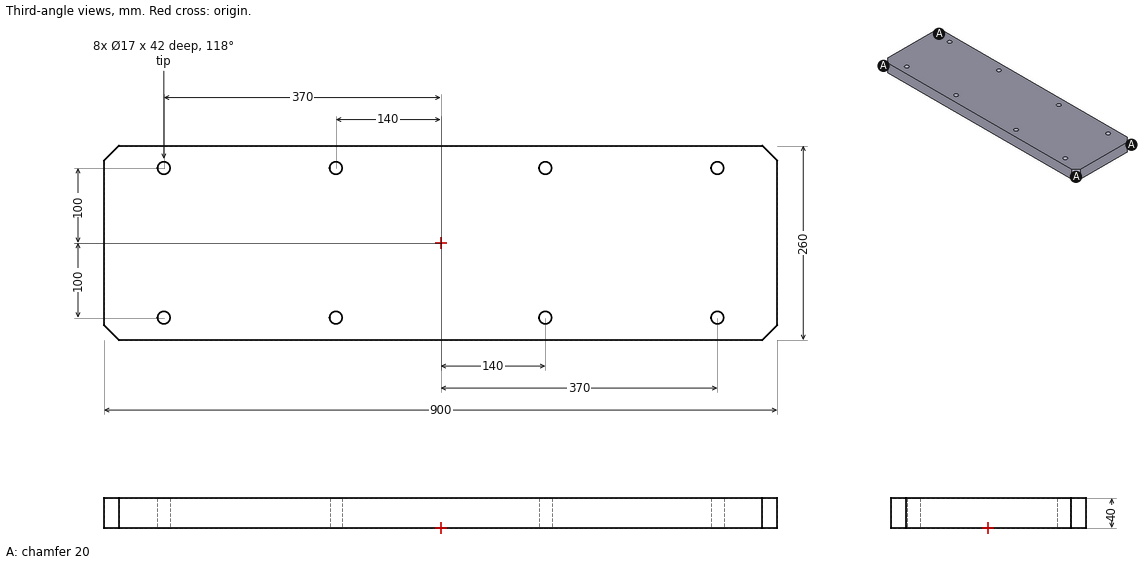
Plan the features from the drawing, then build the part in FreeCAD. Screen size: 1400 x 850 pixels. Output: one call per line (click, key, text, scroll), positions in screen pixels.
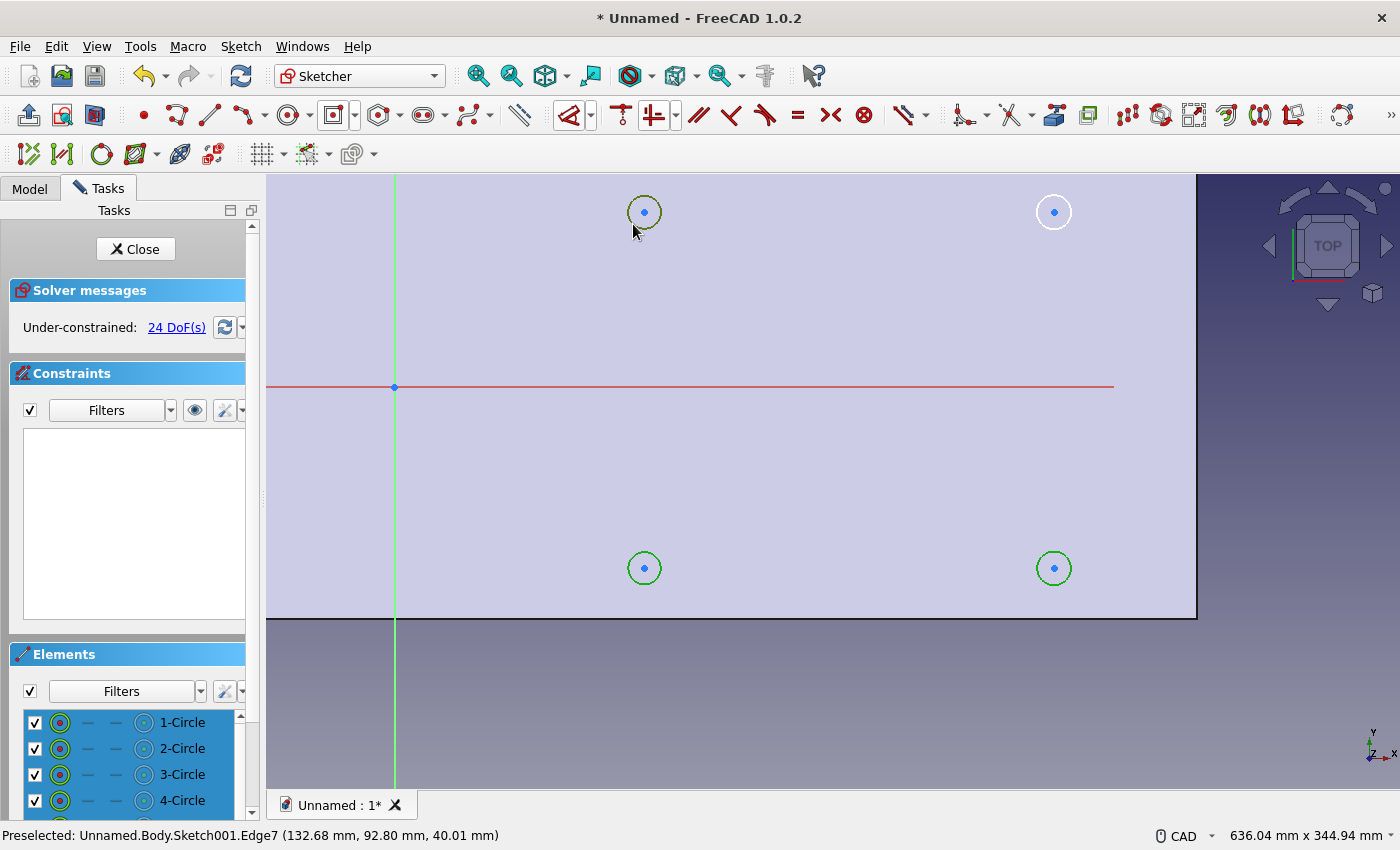
click(1042, 224)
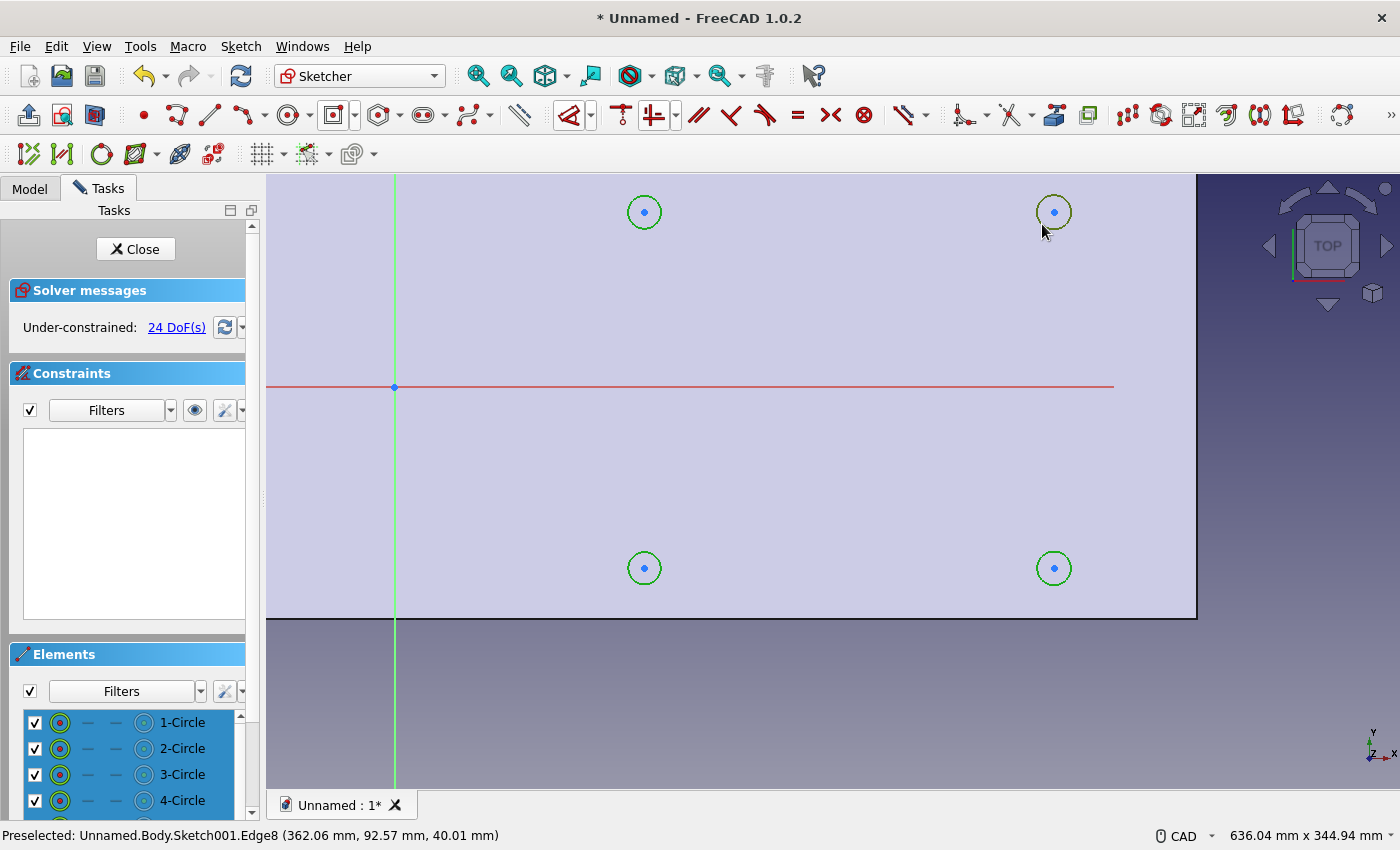
click(798, 116)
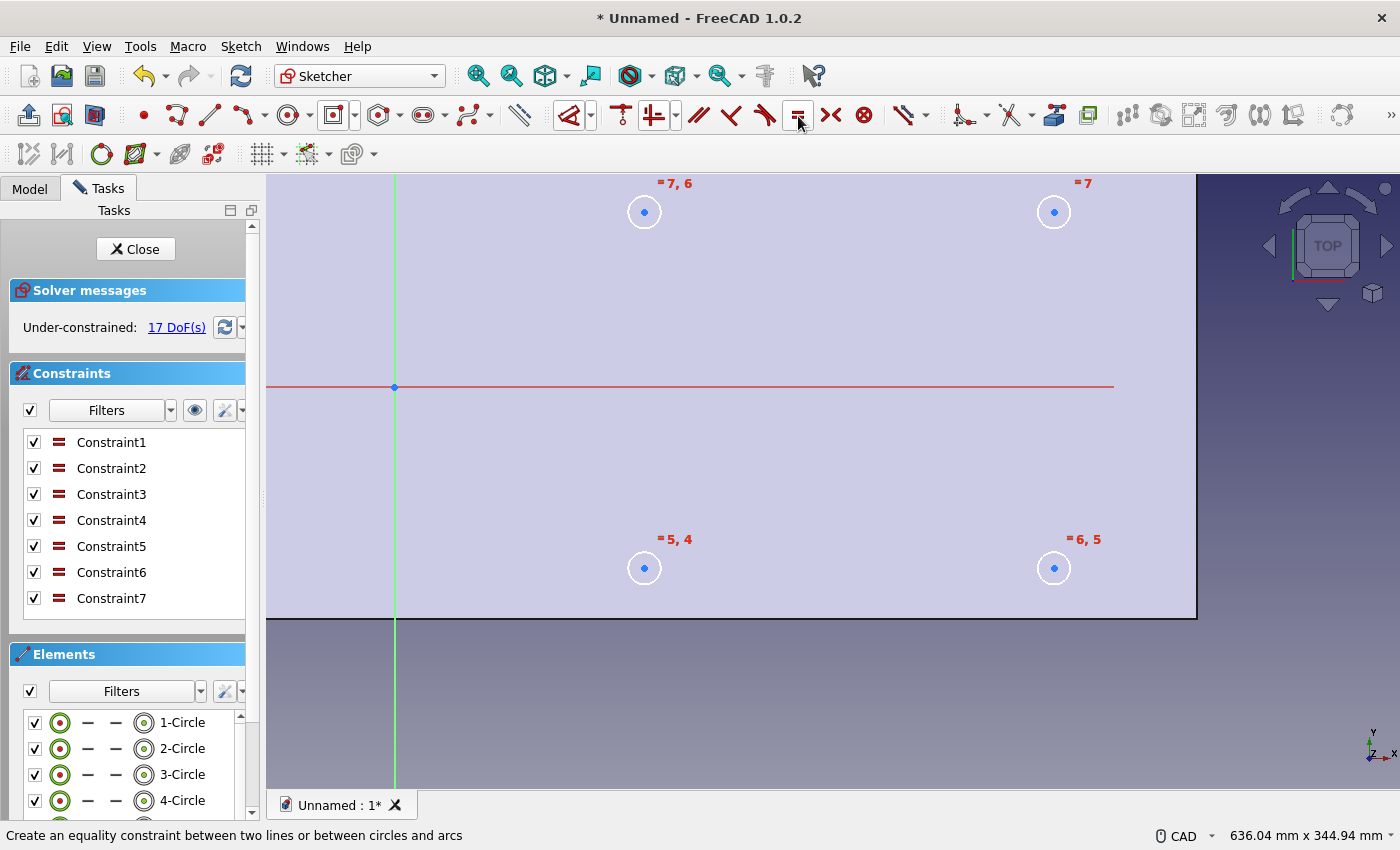
scroll(1066, 558, down, 4)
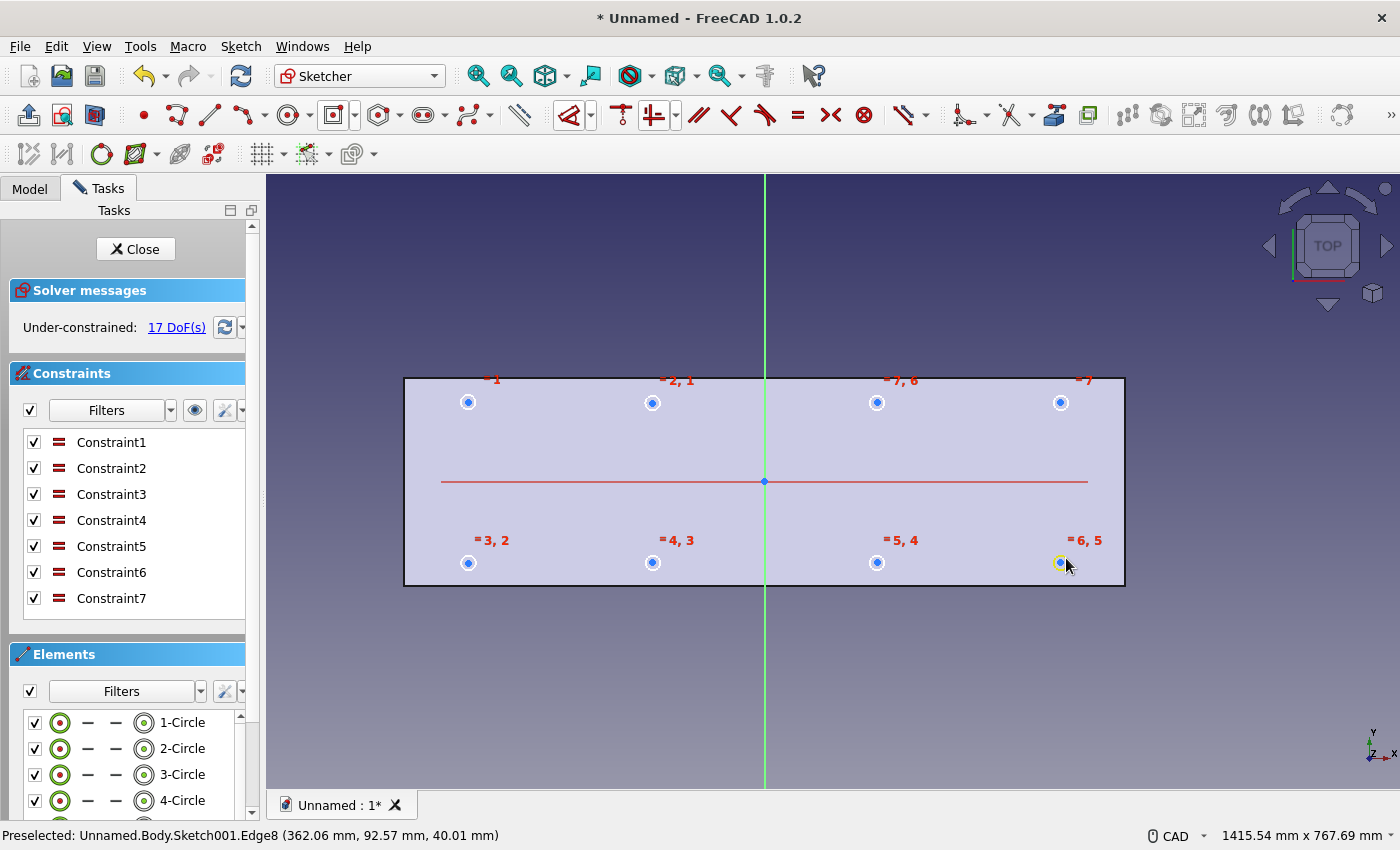
click(468, 402)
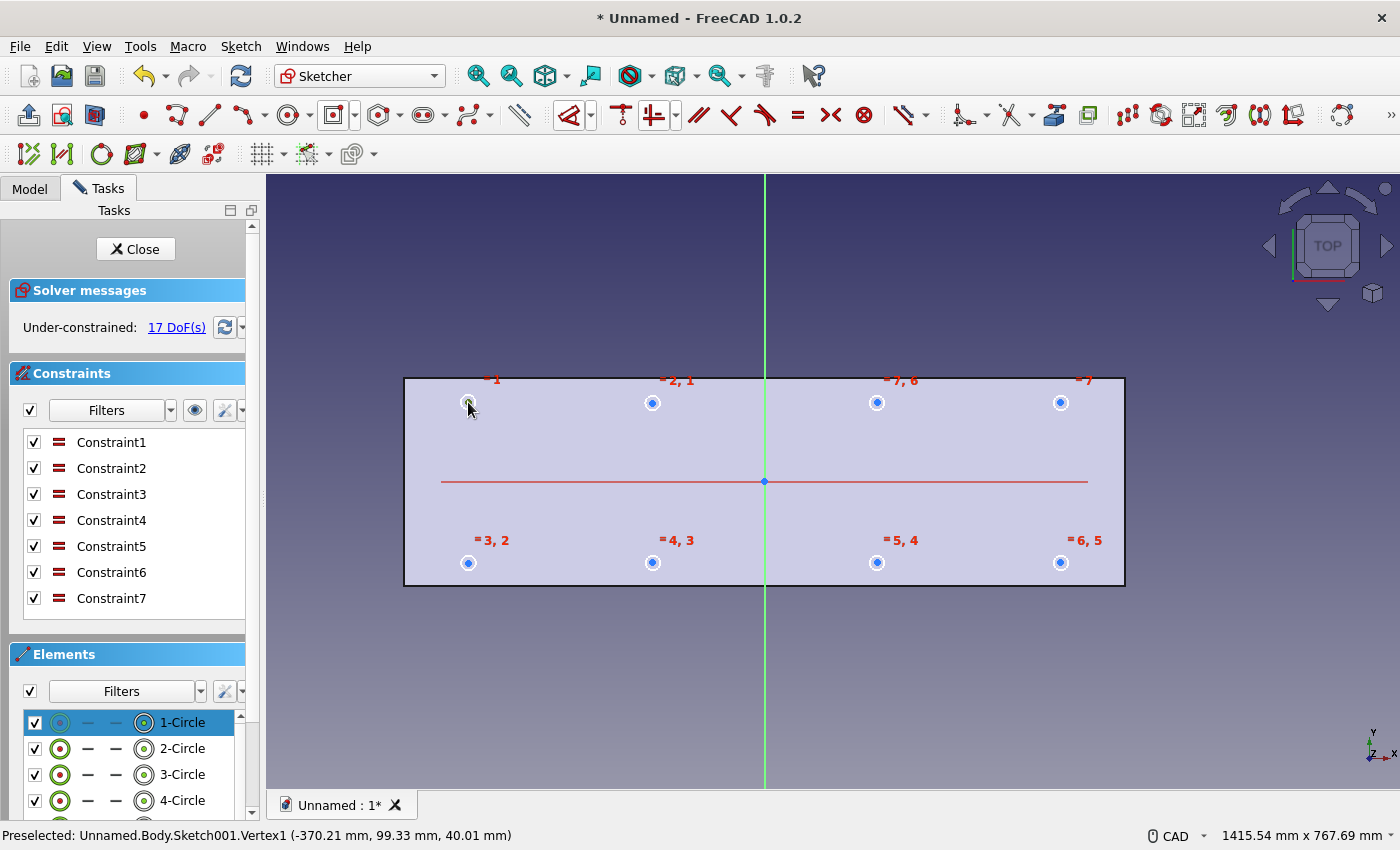
click(653, 403)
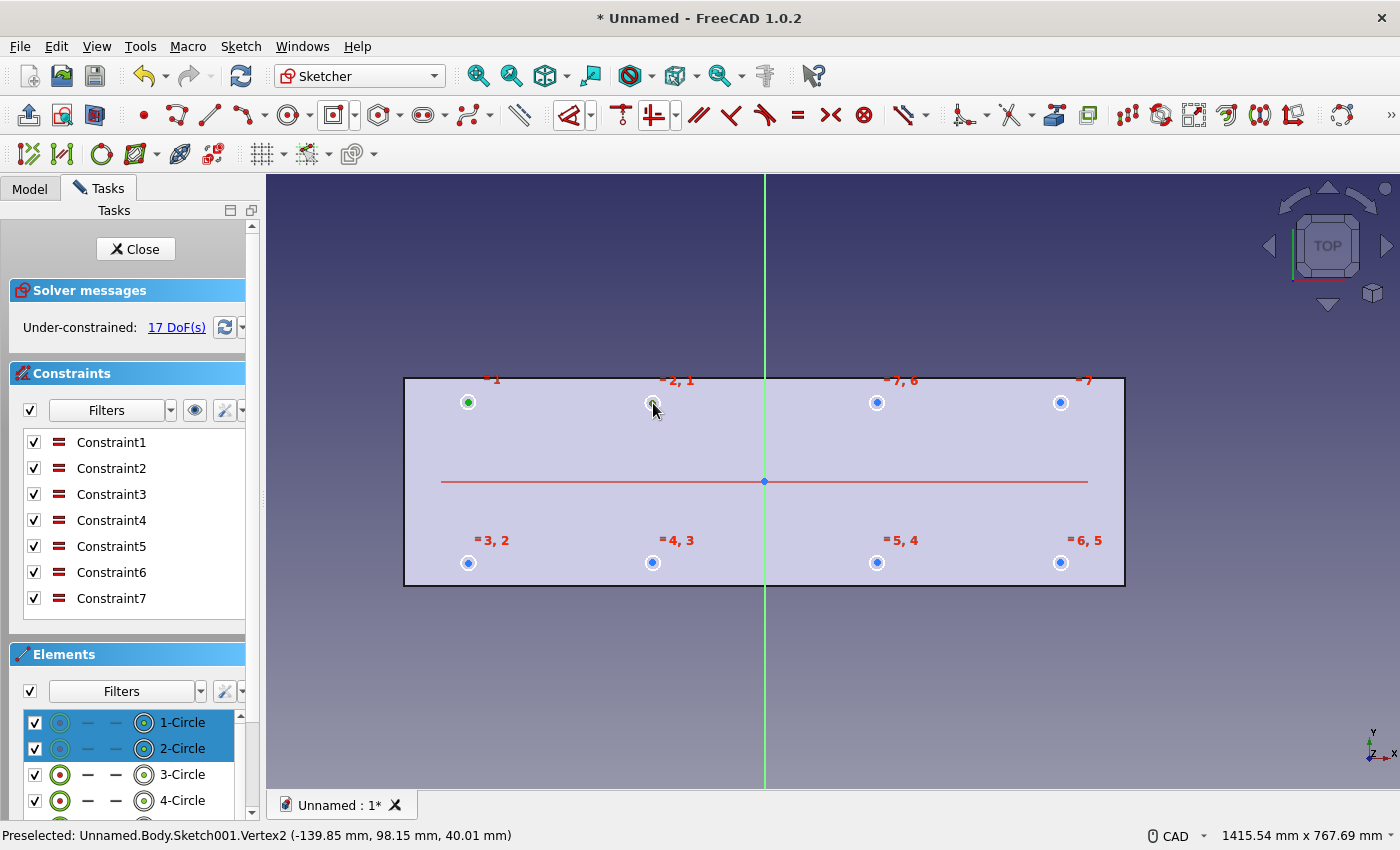
key(h)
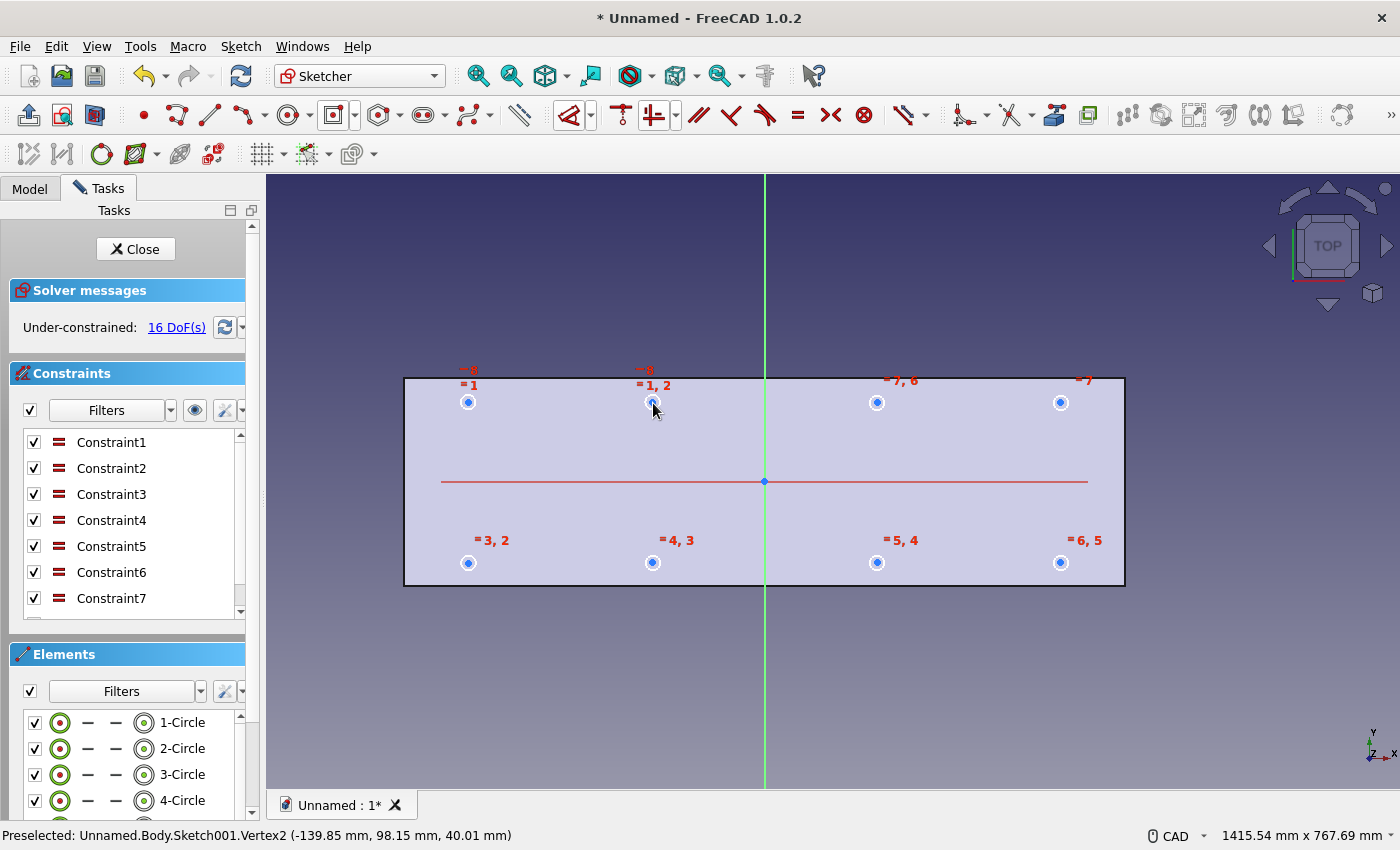
click(468, 402)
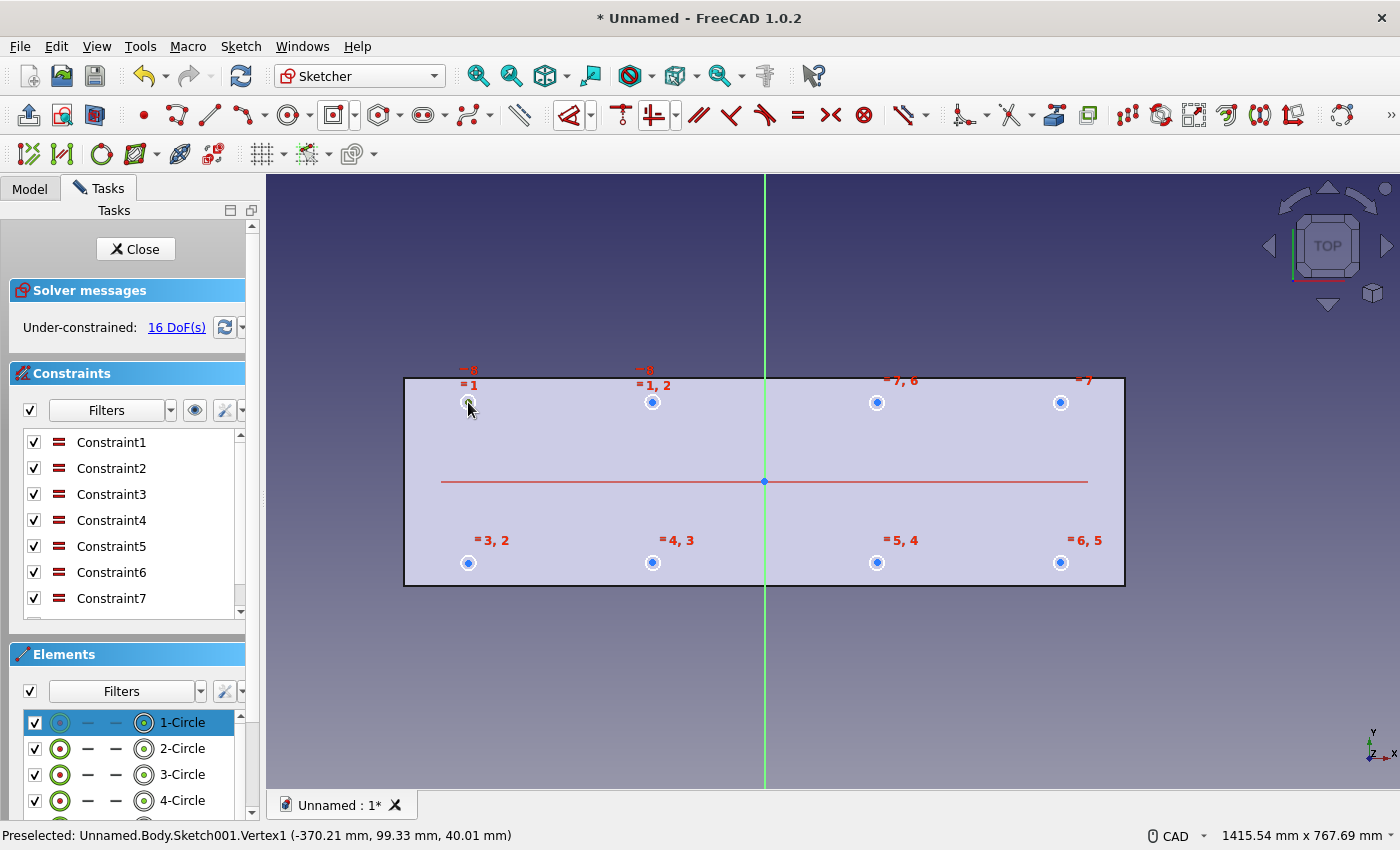
click(468, 563)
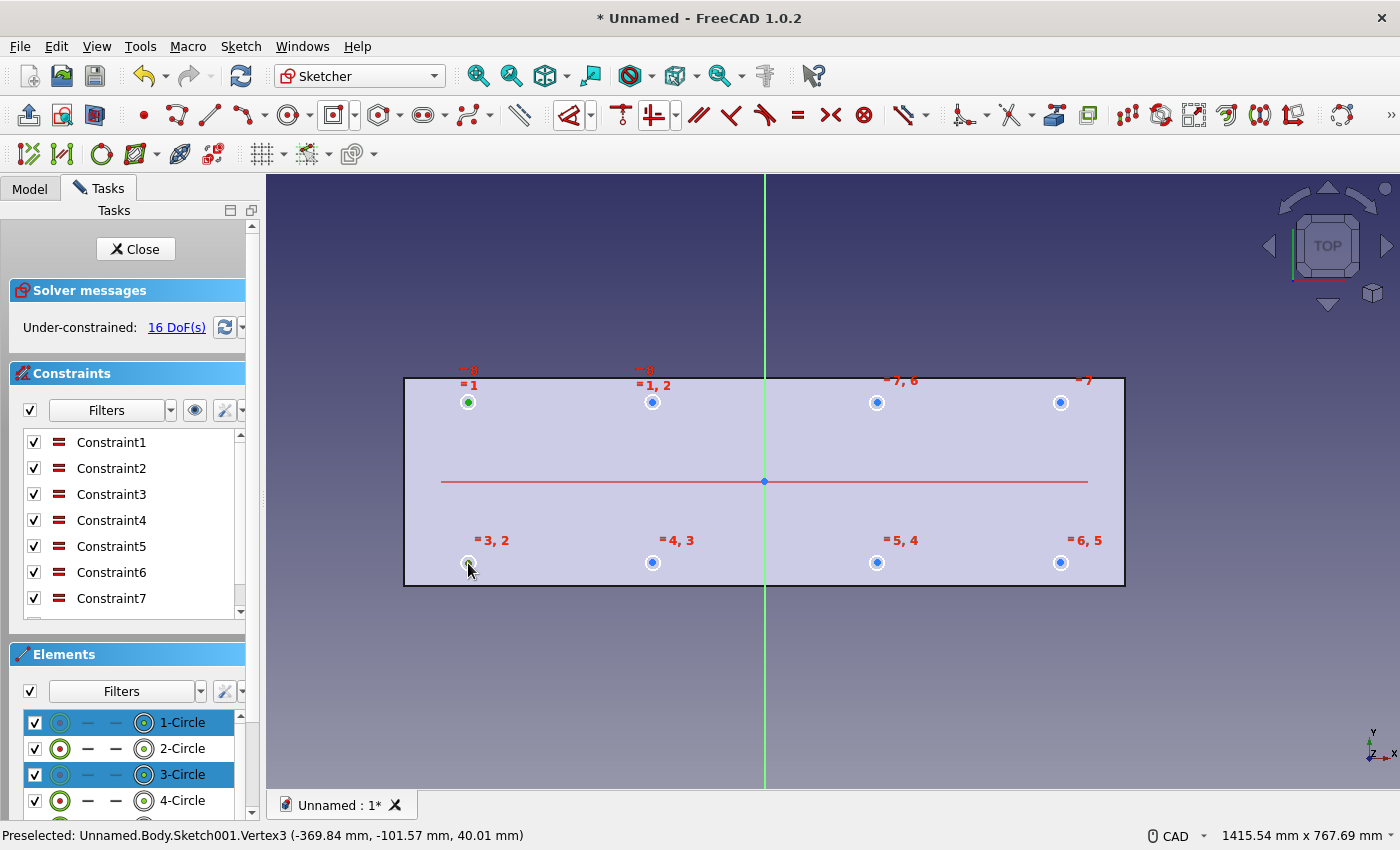
click(676, 116)